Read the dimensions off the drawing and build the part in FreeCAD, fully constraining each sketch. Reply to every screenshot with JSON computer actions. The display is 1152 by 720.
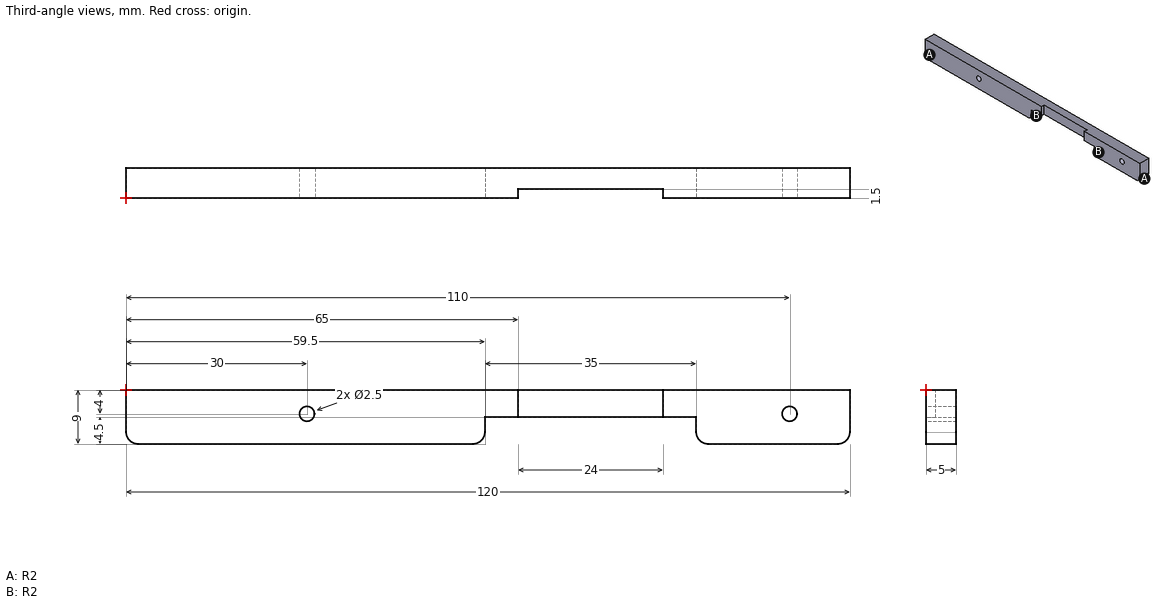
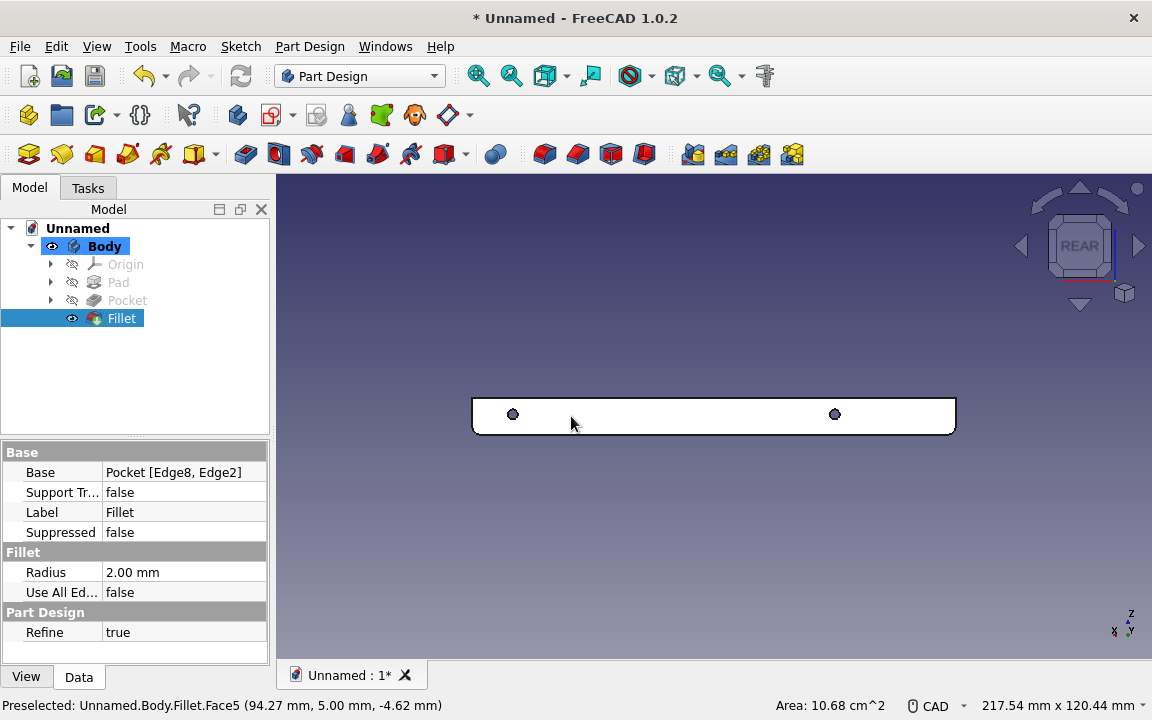
{"action": "left_click", "coordinate": [270, 116]}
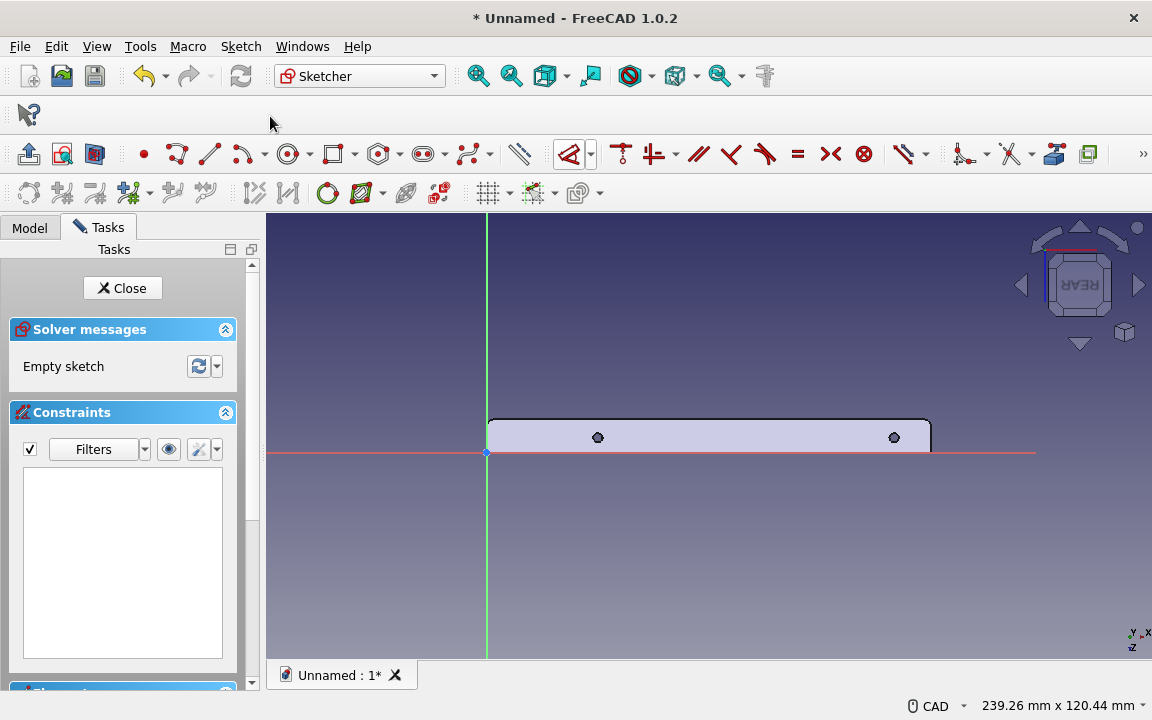
{"action": "scroll", "coordinate": [815, 425], "scroll_direction": "up", "scroll_amount": 7}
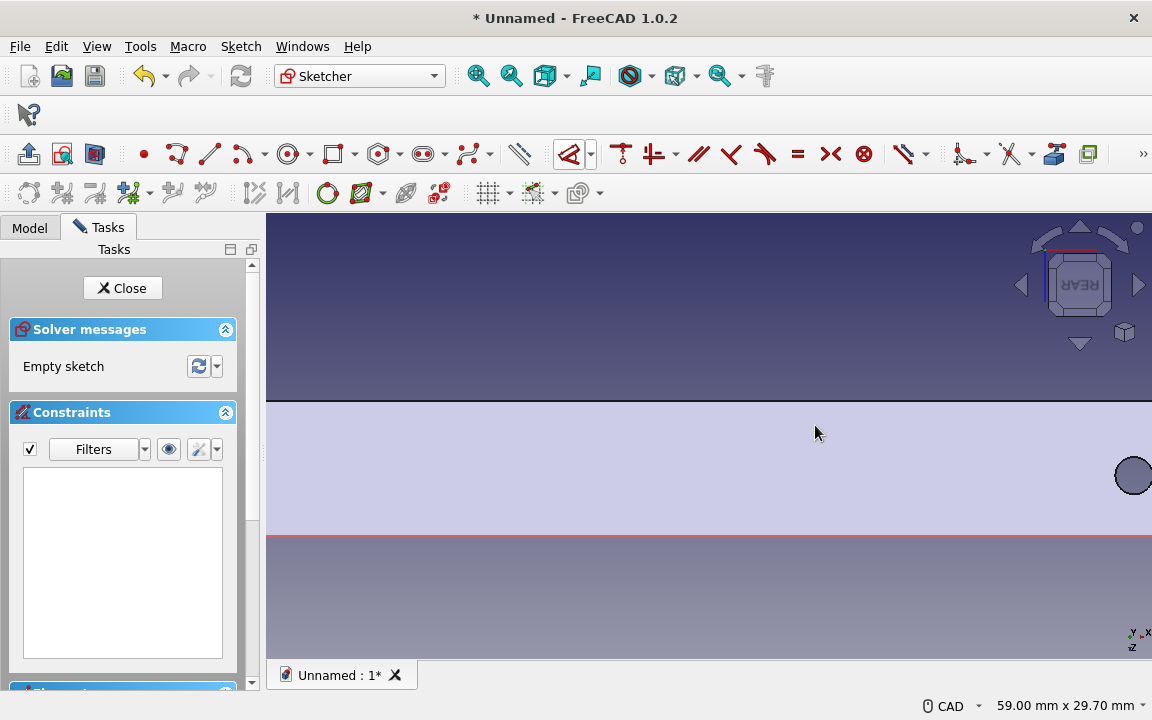
{"action": "key", "text": "g r"}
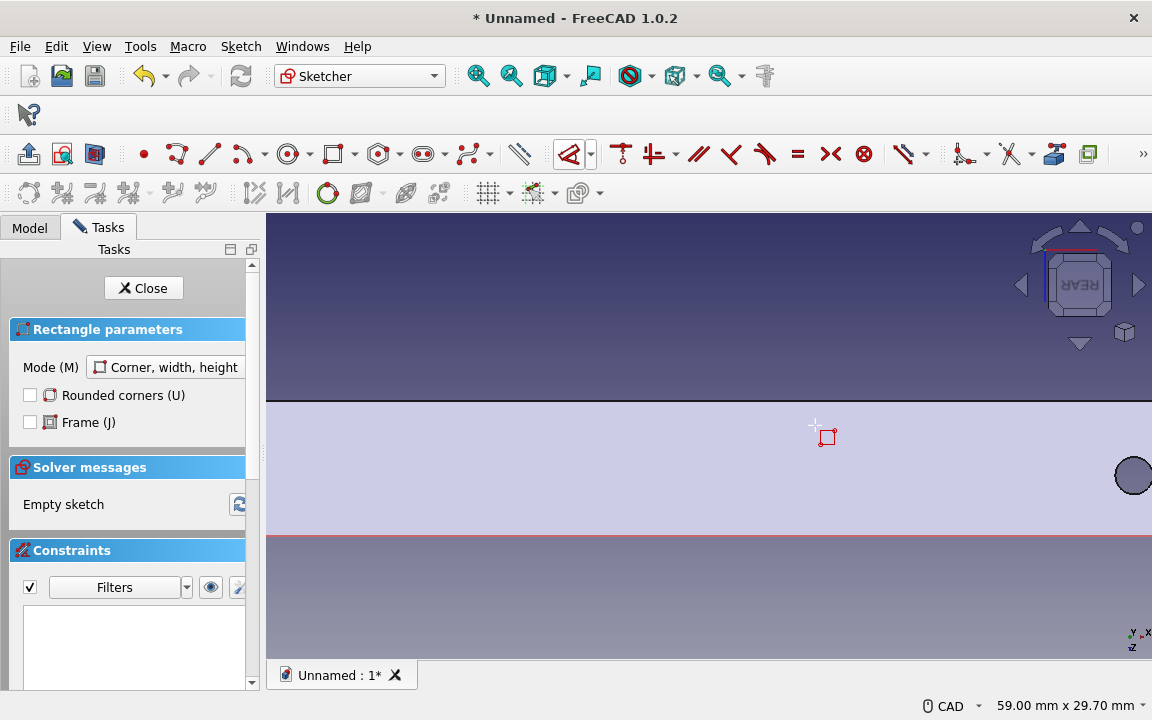
{"action": "left_click", "coordinate": [376, 401]}
{"action": "left_click", "coordinate": [901, 468]}
{"action": "key", "text": "Escape"}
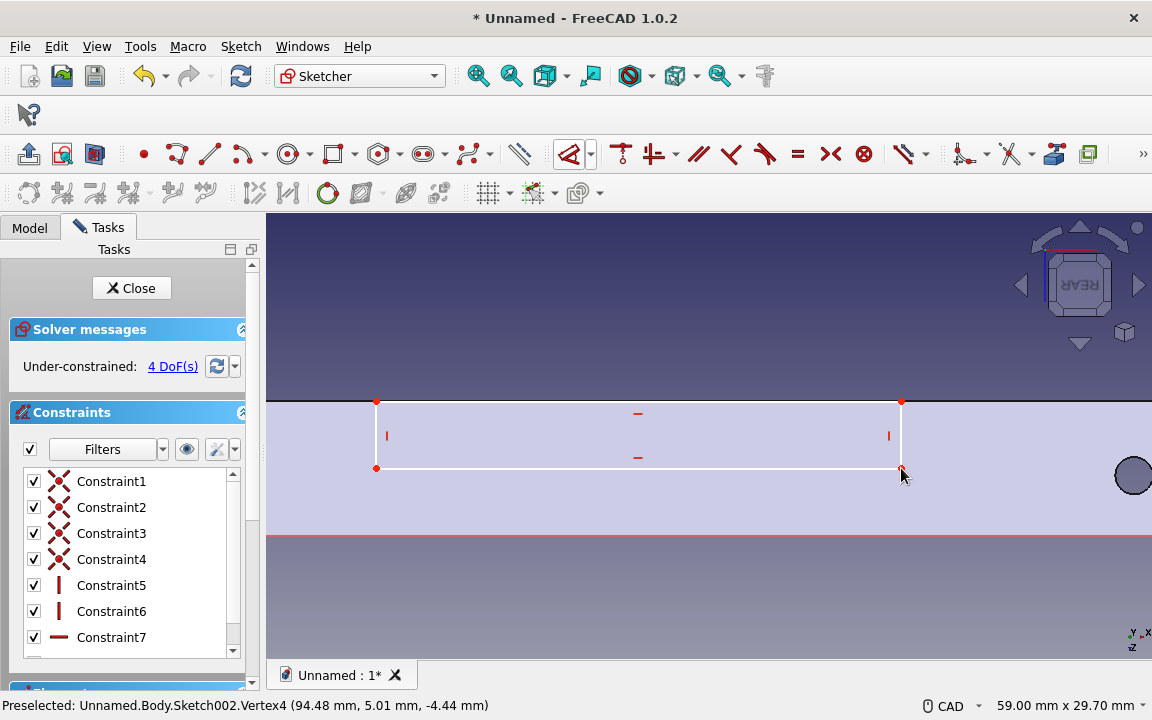
{"action": "key", "text": "d"}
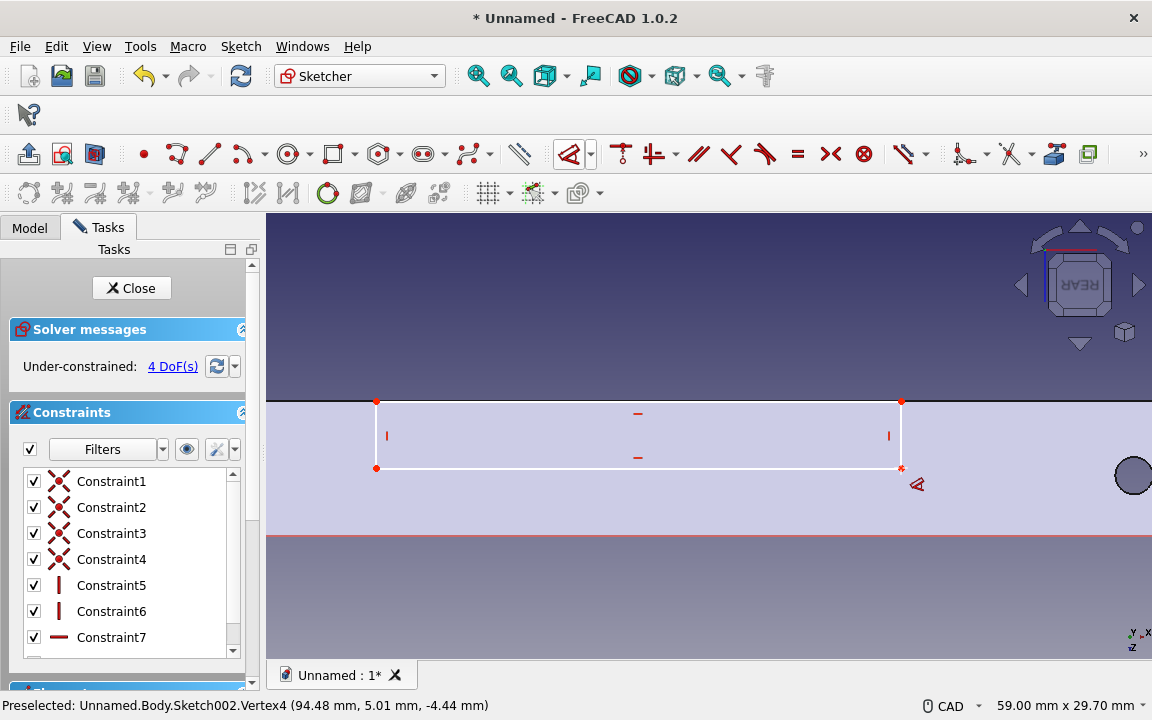
{"action": "left_click", "coordinate": [534, 469]}
{"action": "left_click", "coordinate": [639, 503]}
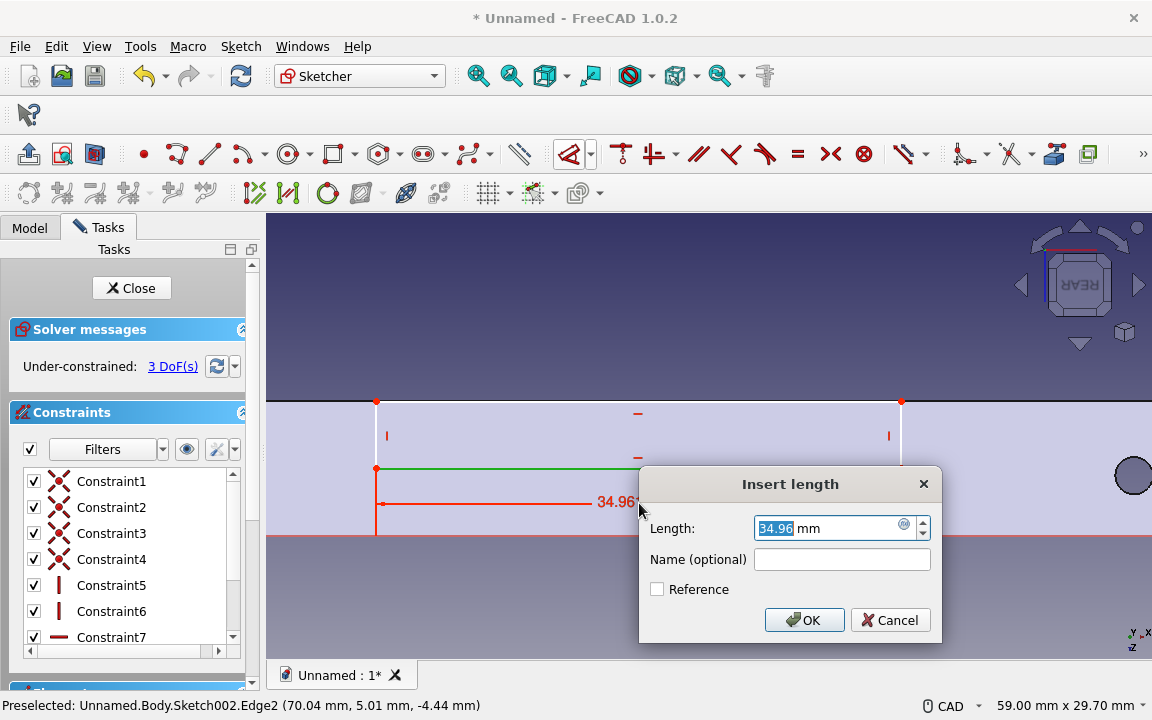
{"action": "type", "text": "35"}
{"action": "key", "text": "Return"}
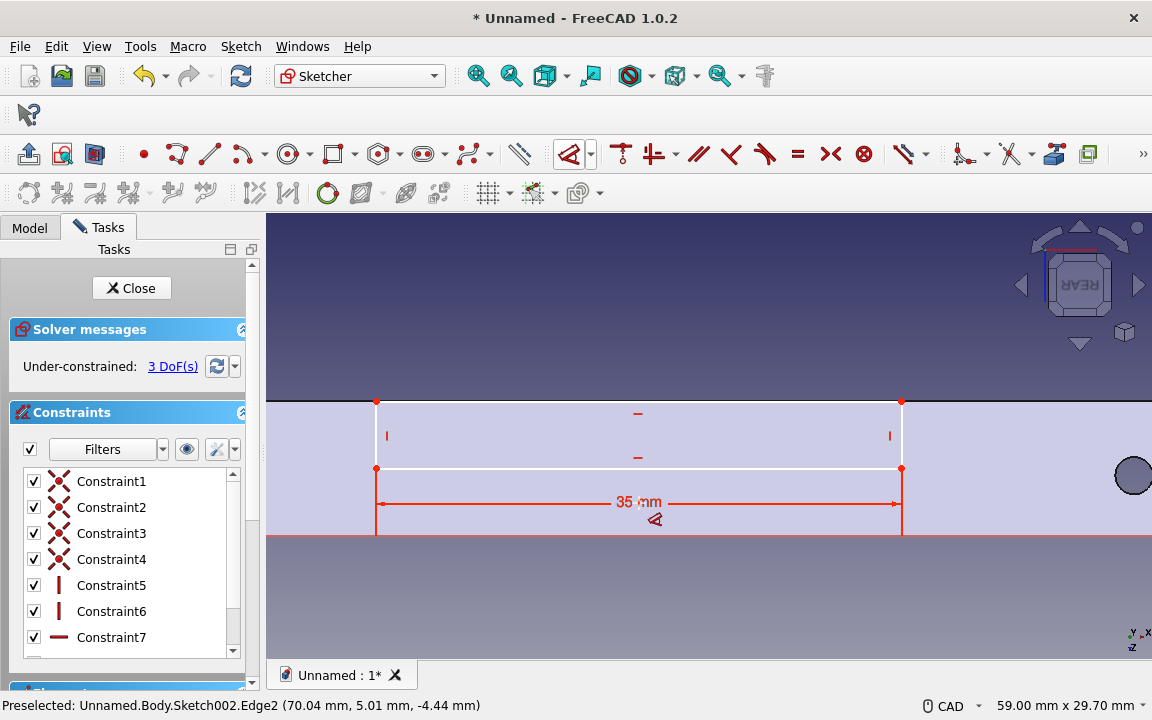
{"action": "left_click", "coordinate": [376, 402]}
{"action": "left_click", "coordinate": [410, 438]}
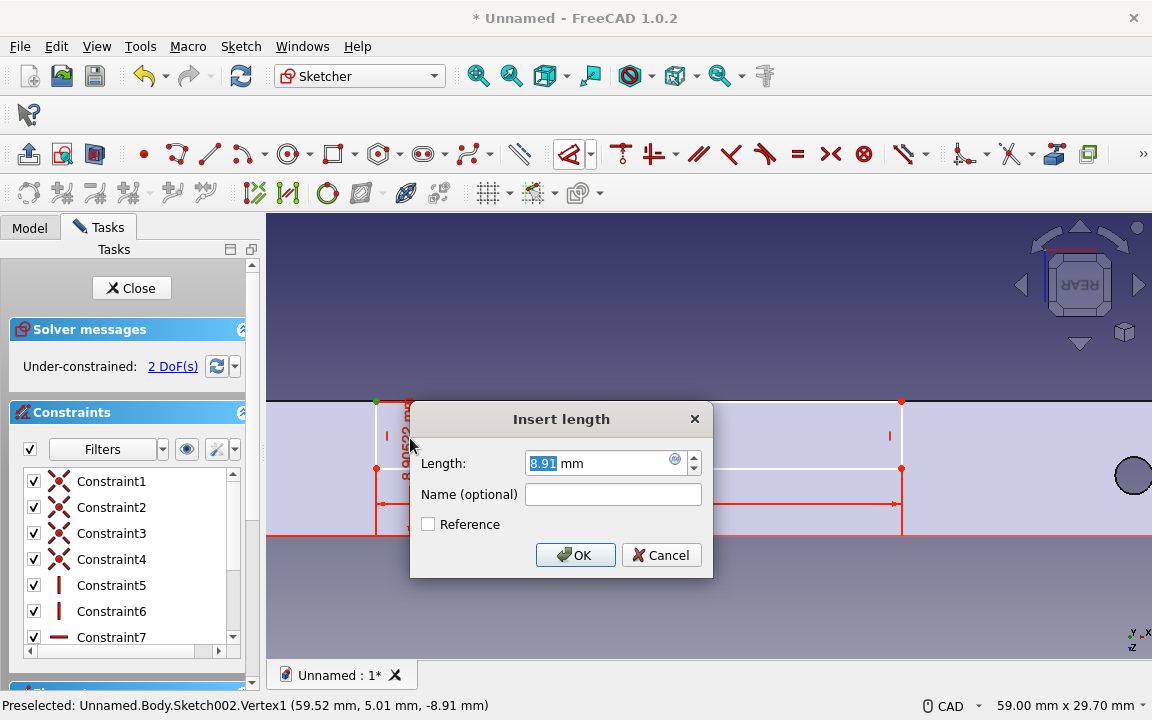
{"action": "type", "text": "9"}
{"action": "key", "text": "Return"}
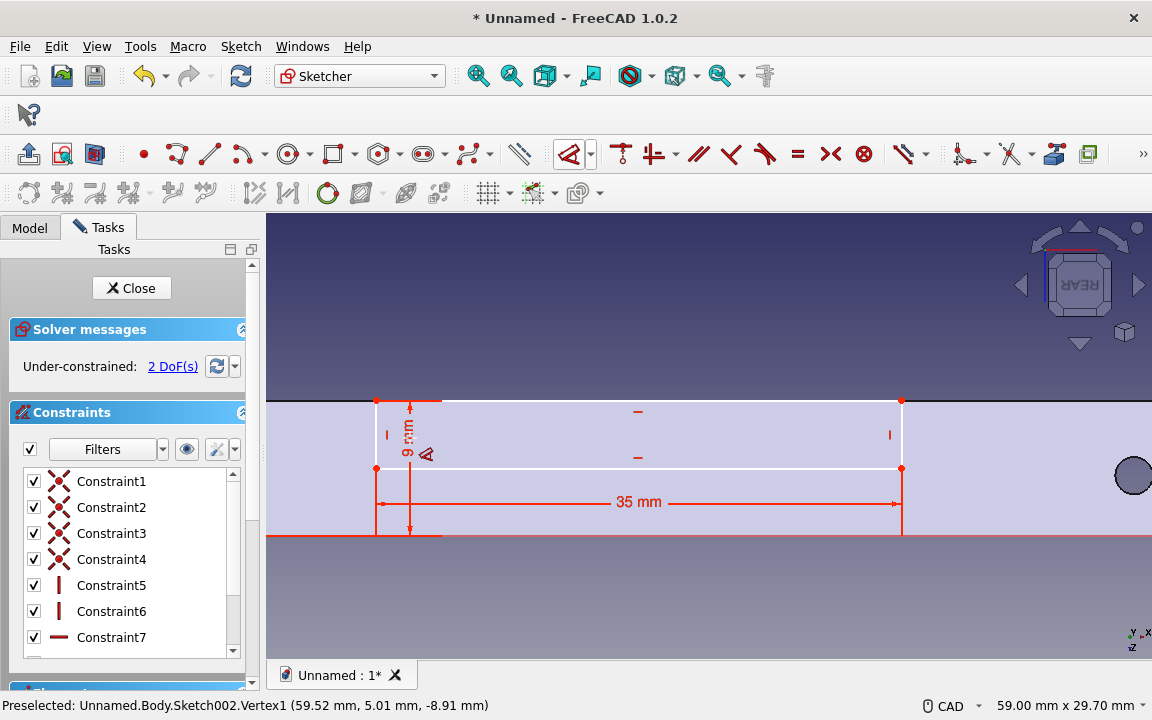
{"action": "left_click", "coordinate": [376, 421]}
{"action": "left_click", "coordinate": [342, 411]}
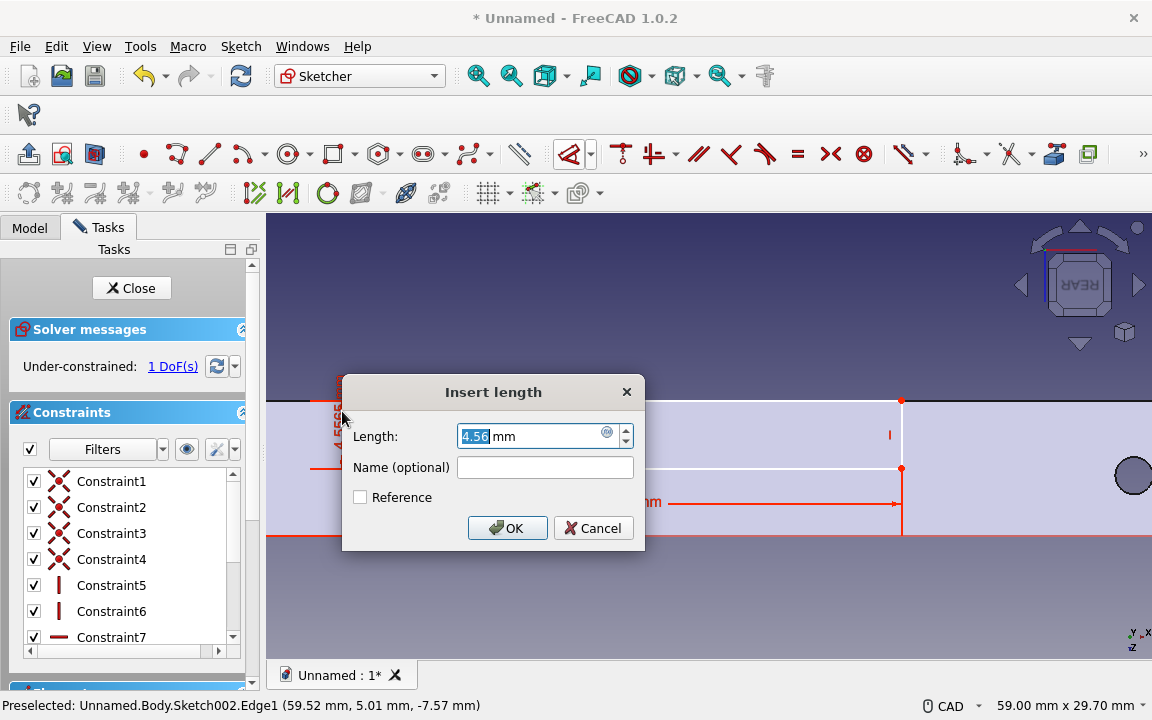
{"action": "type", "text": "4.5"}
{"action": "key", "text": "Return"}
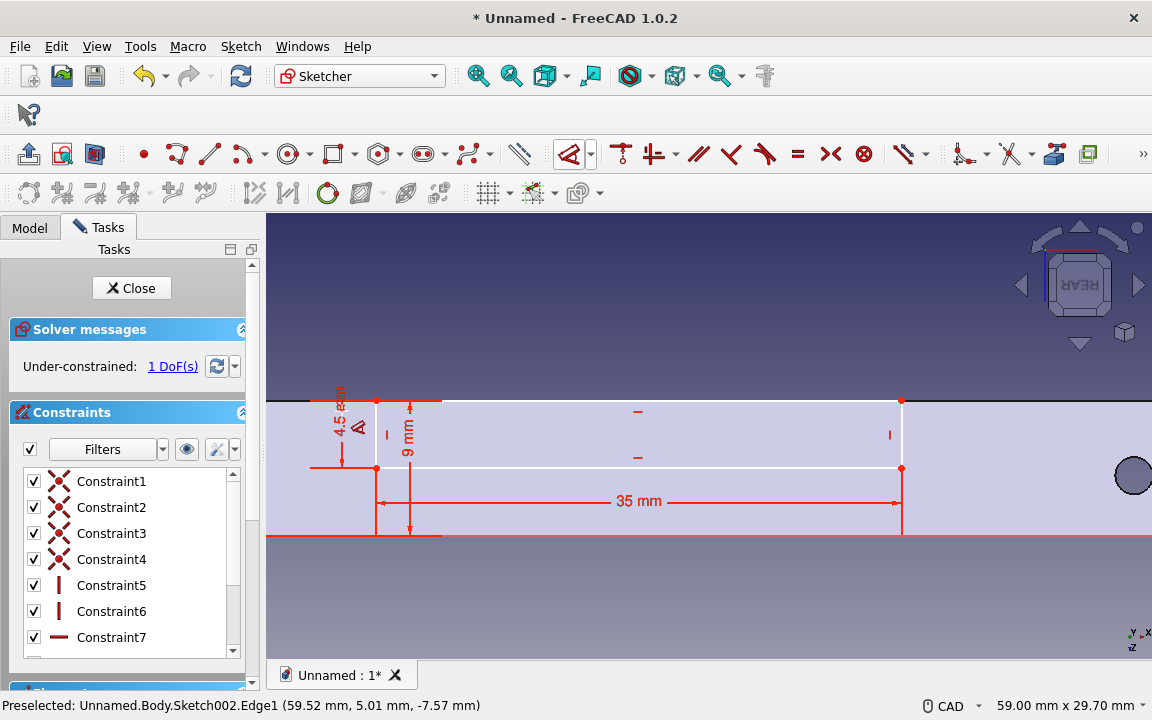
{"action": "left_click", "coordinate": [376, 401]}
{"action": "left_click", "coordinate": [335, 570]}